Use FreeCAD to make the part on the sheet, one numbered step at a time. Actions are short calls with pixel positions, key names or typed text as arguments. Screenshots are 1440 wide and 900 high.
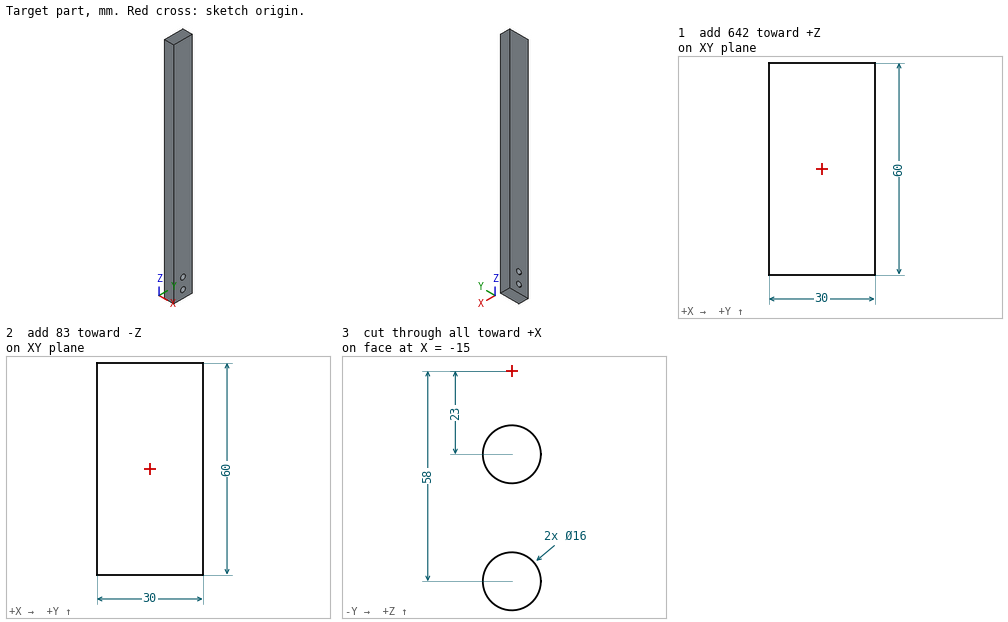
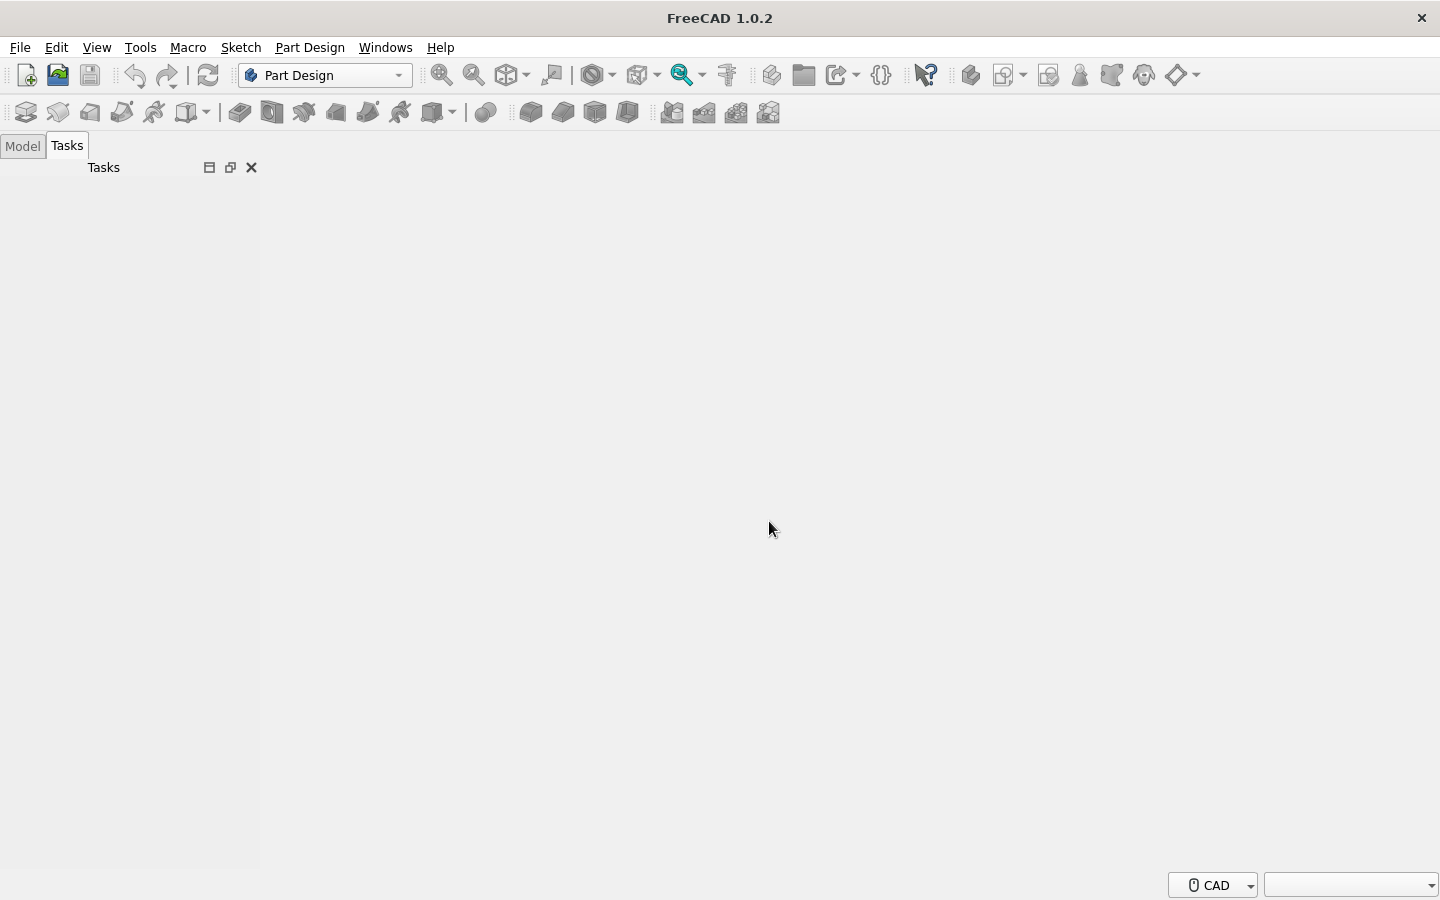
click(26, 76)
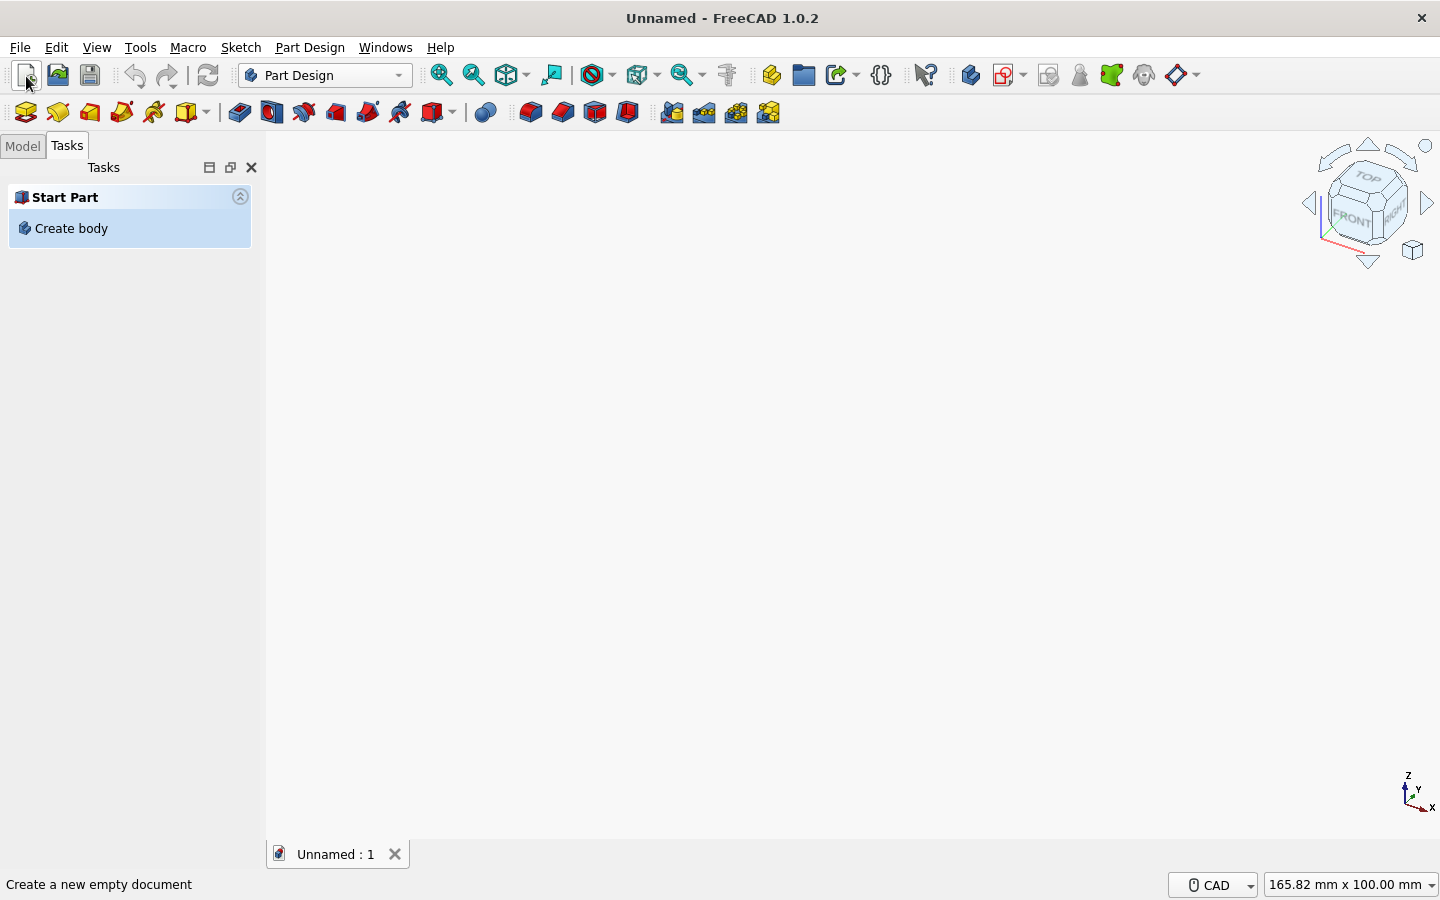
click(1004, 76)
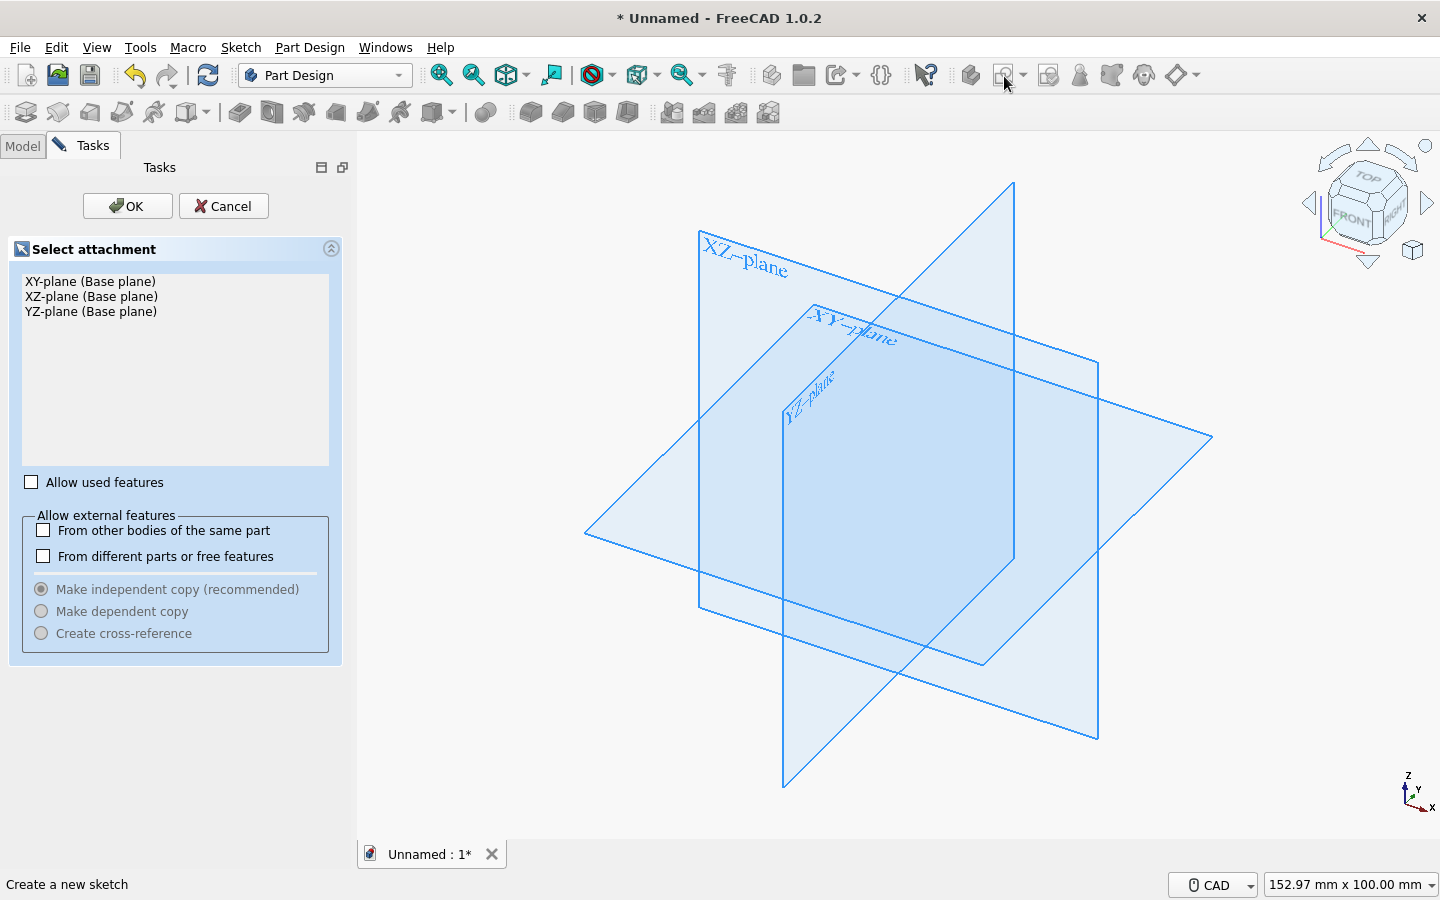
click(82, 282)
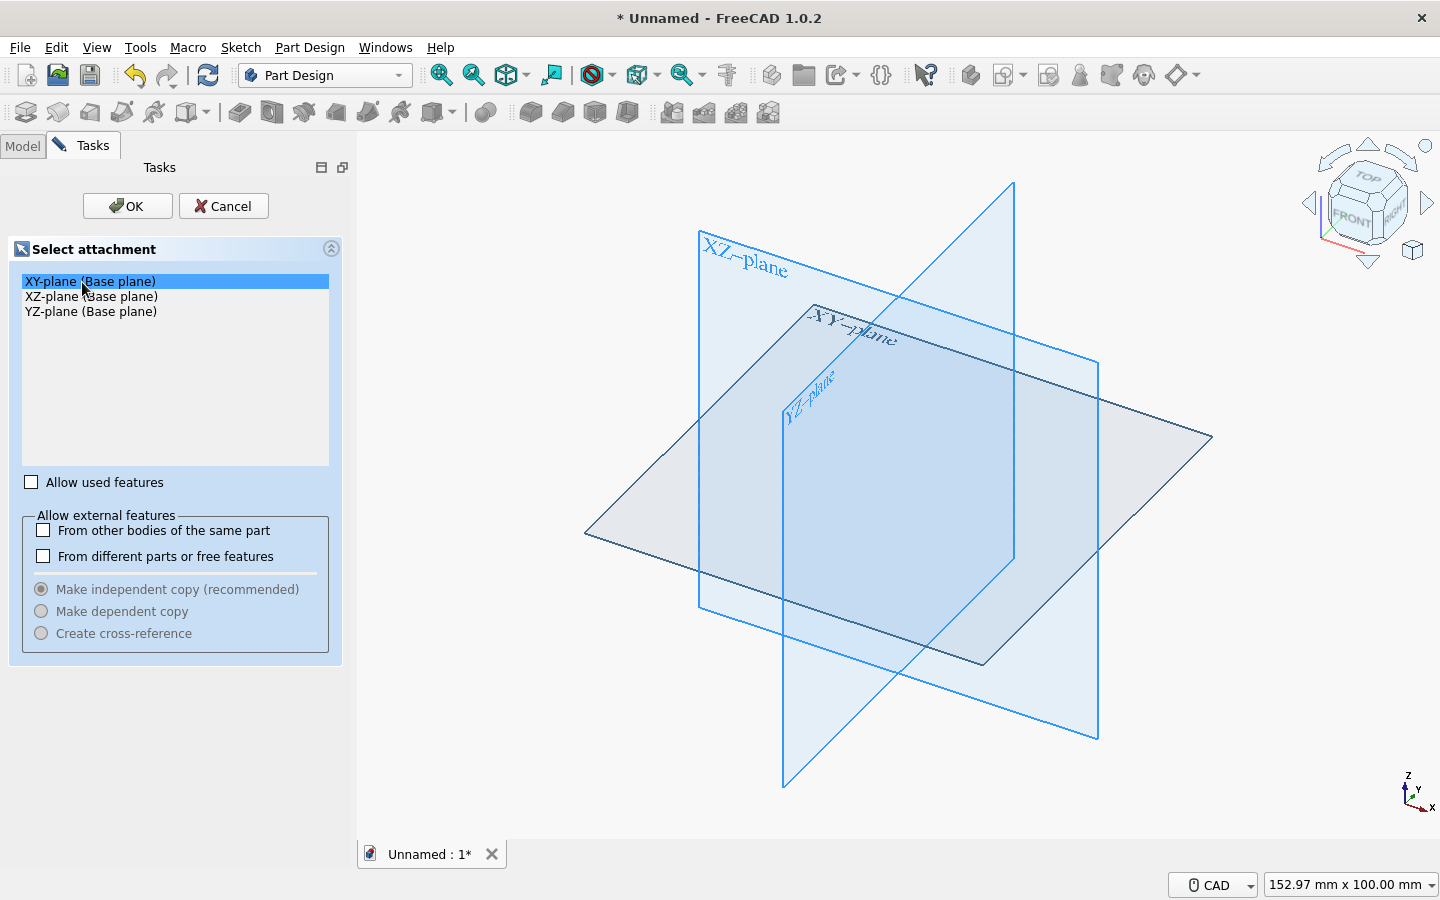
click(128, 206)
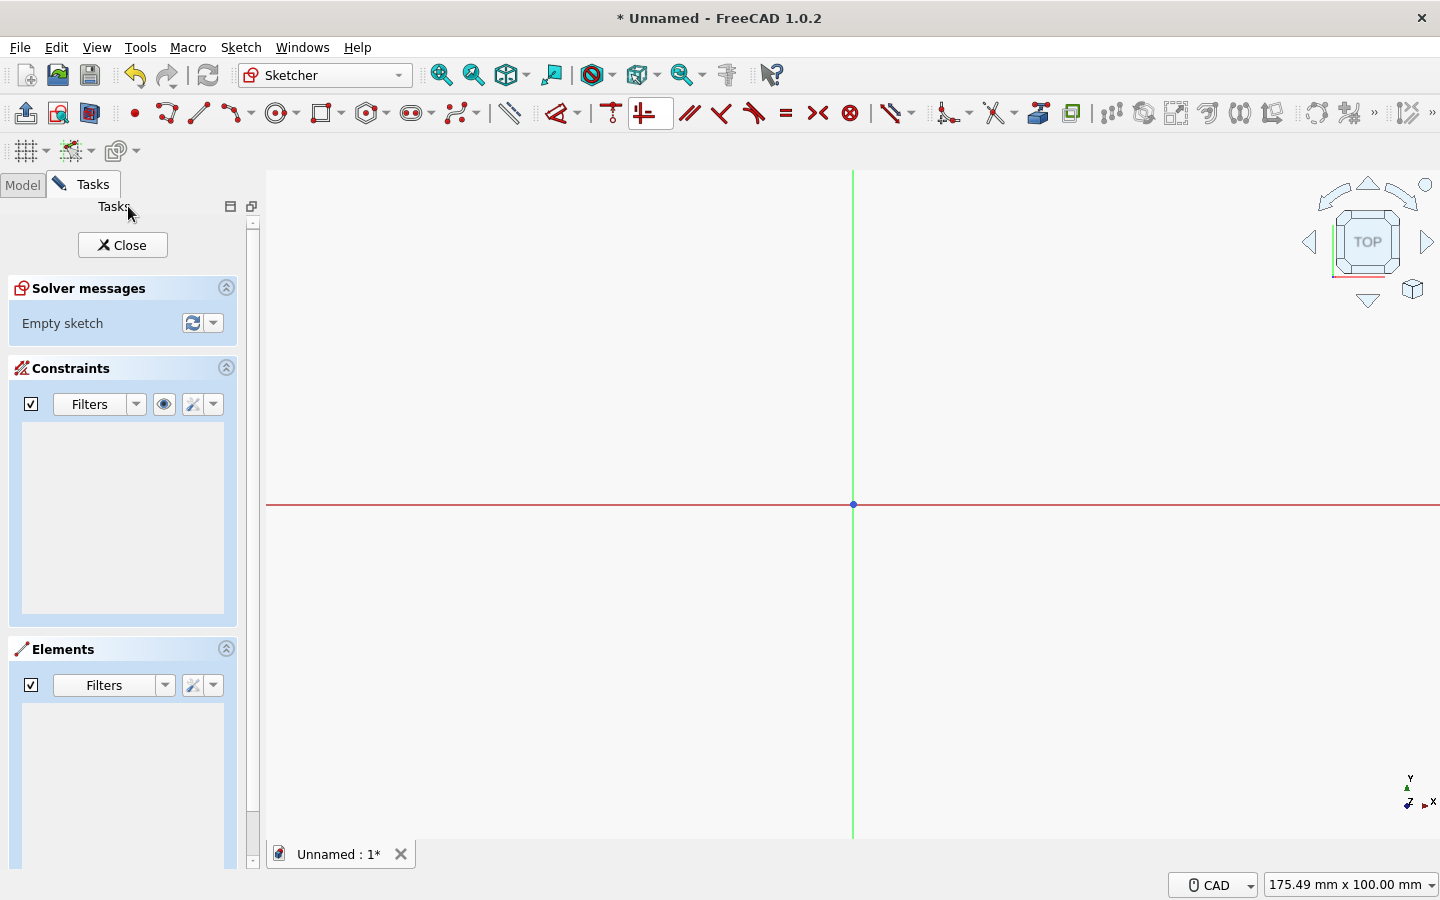
key(g)
key(v)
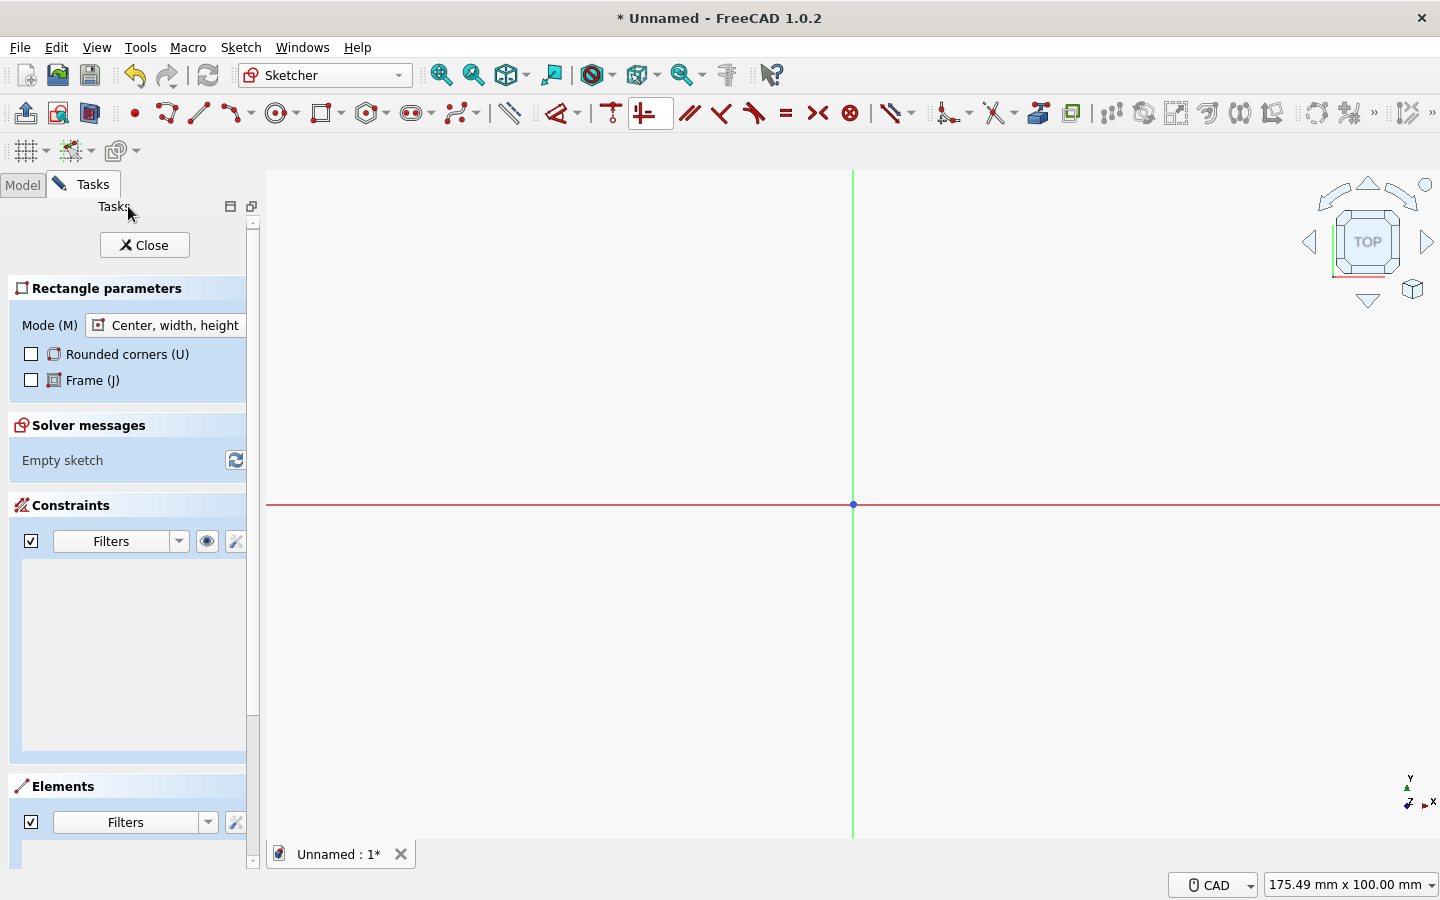
click(853, 504)
move(953, 304)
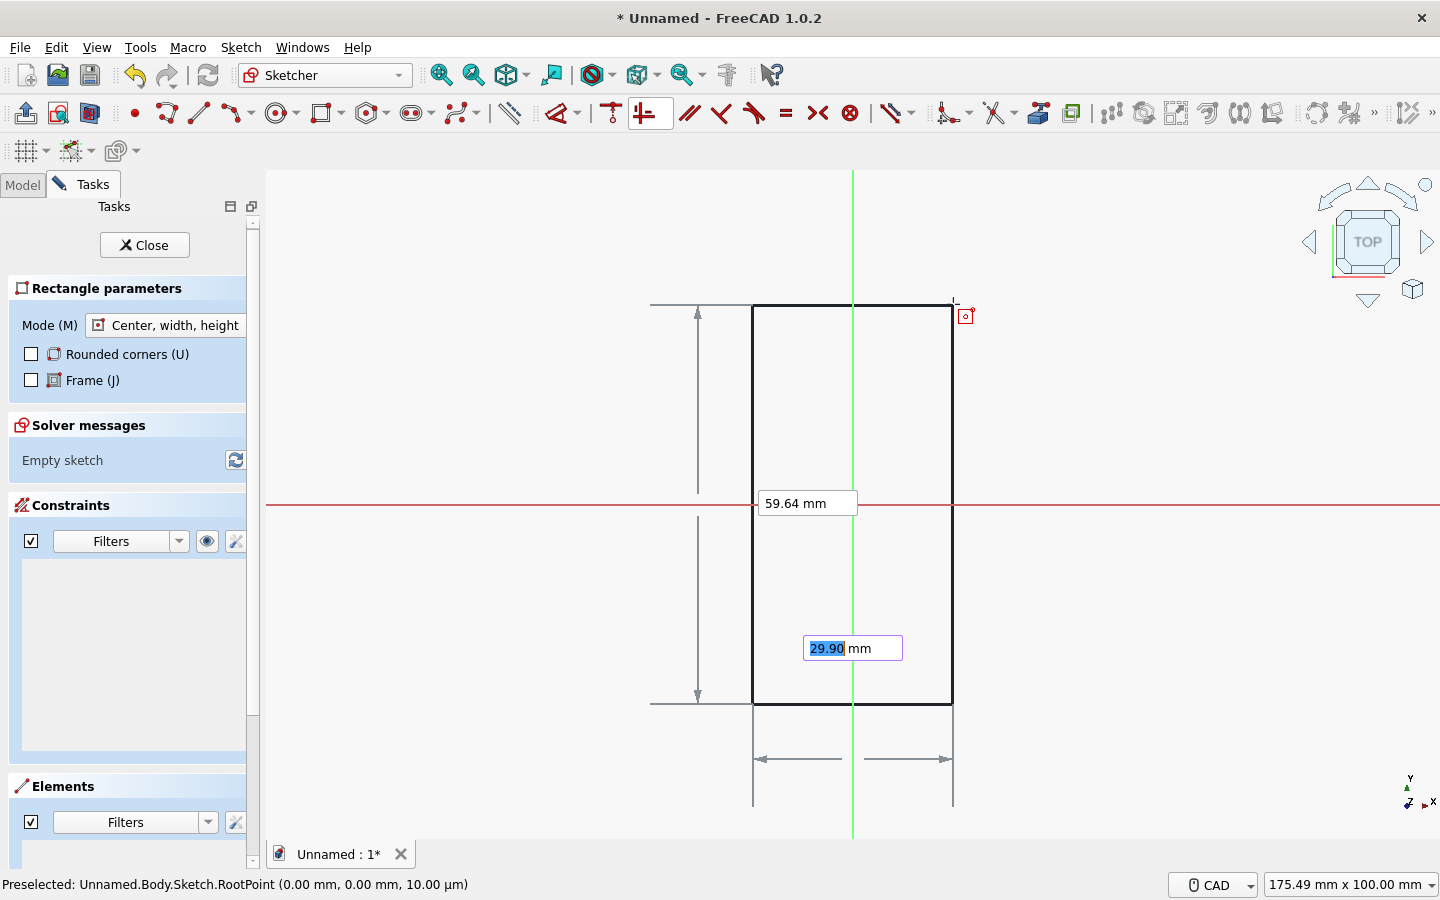
text(30)
key(Tab)
text(60)
key(Return)
key(Escape)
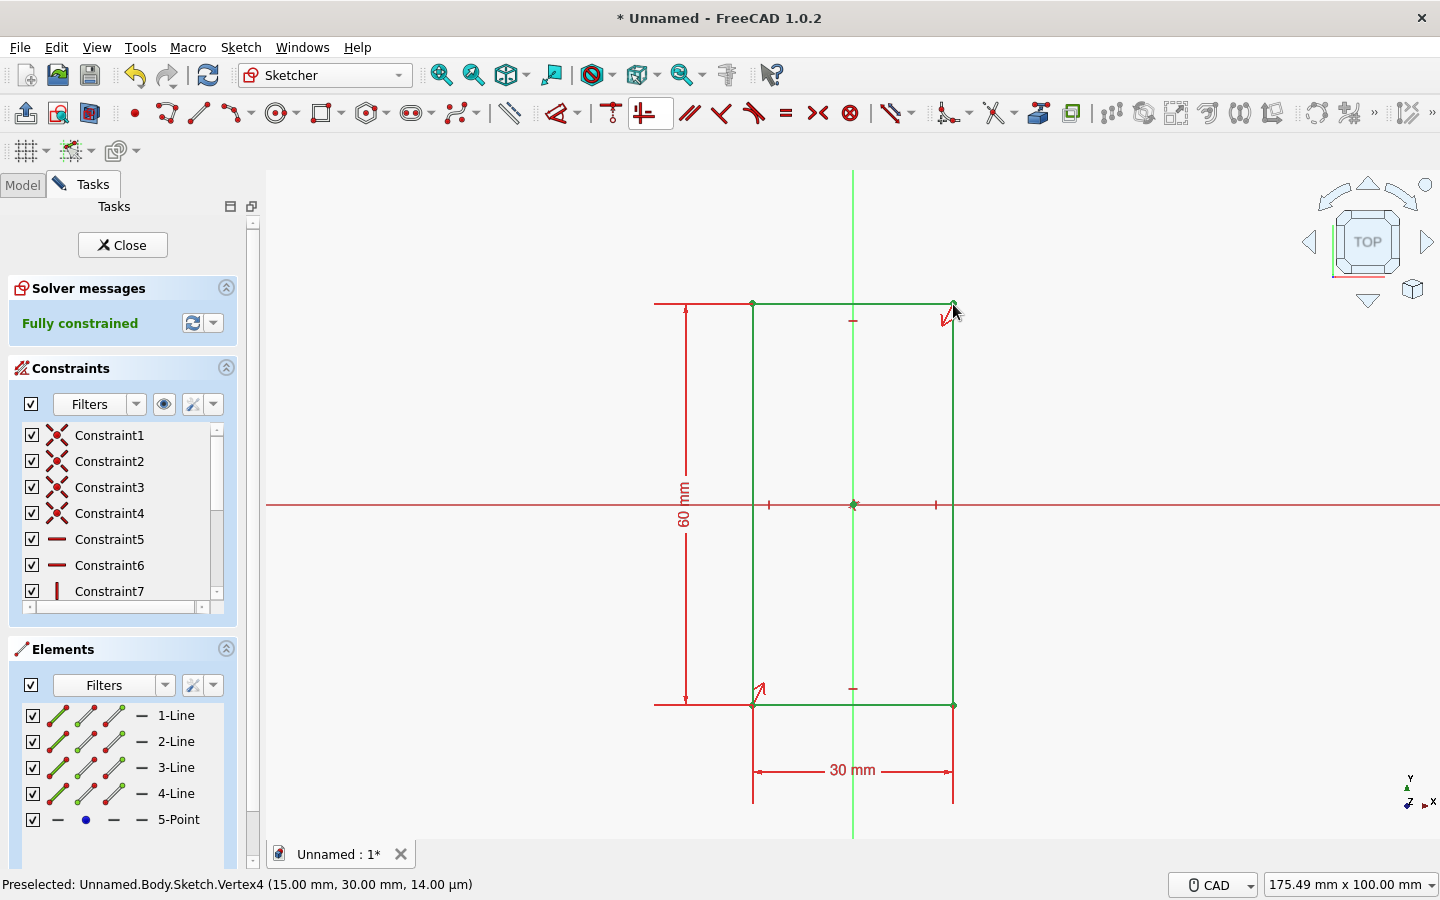
click(123, 245)